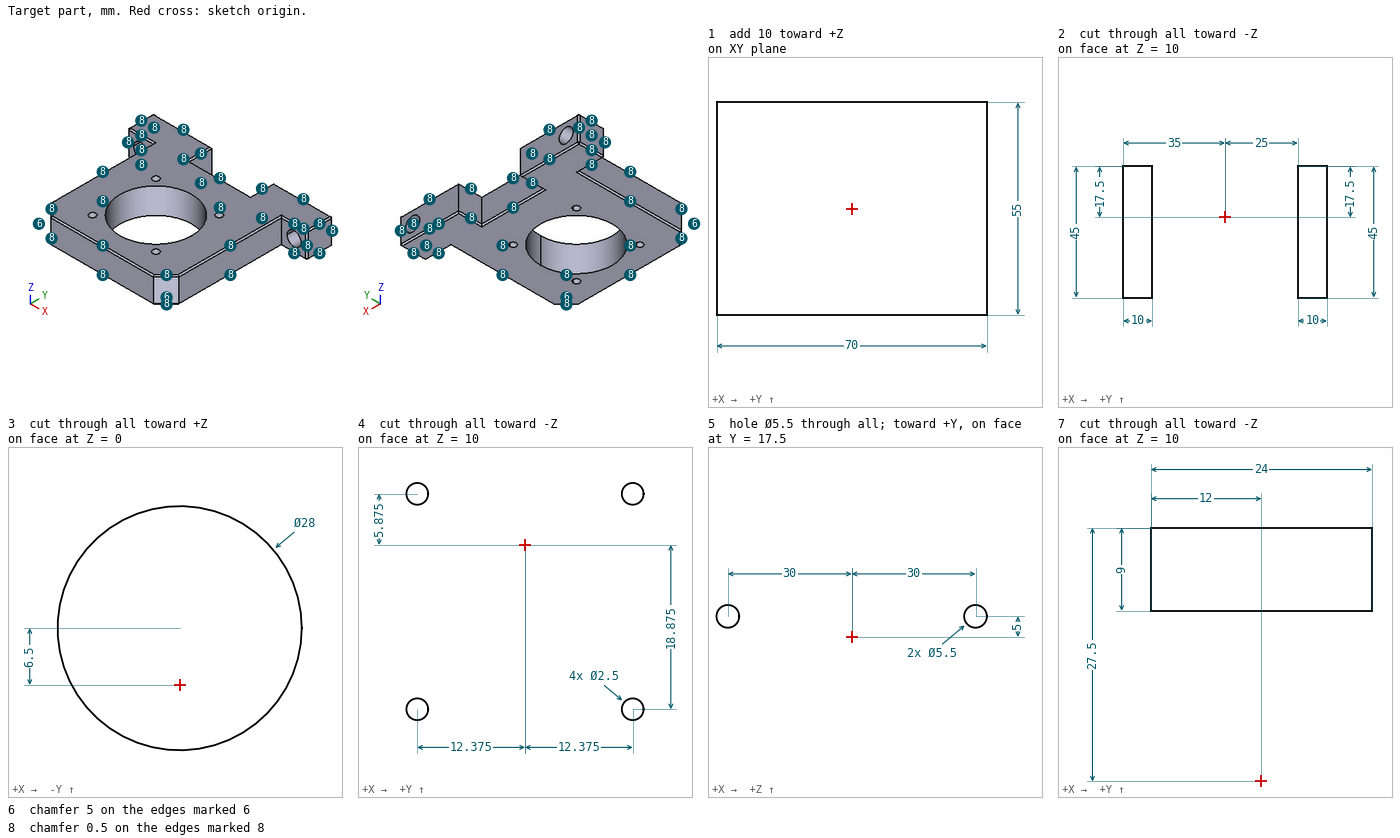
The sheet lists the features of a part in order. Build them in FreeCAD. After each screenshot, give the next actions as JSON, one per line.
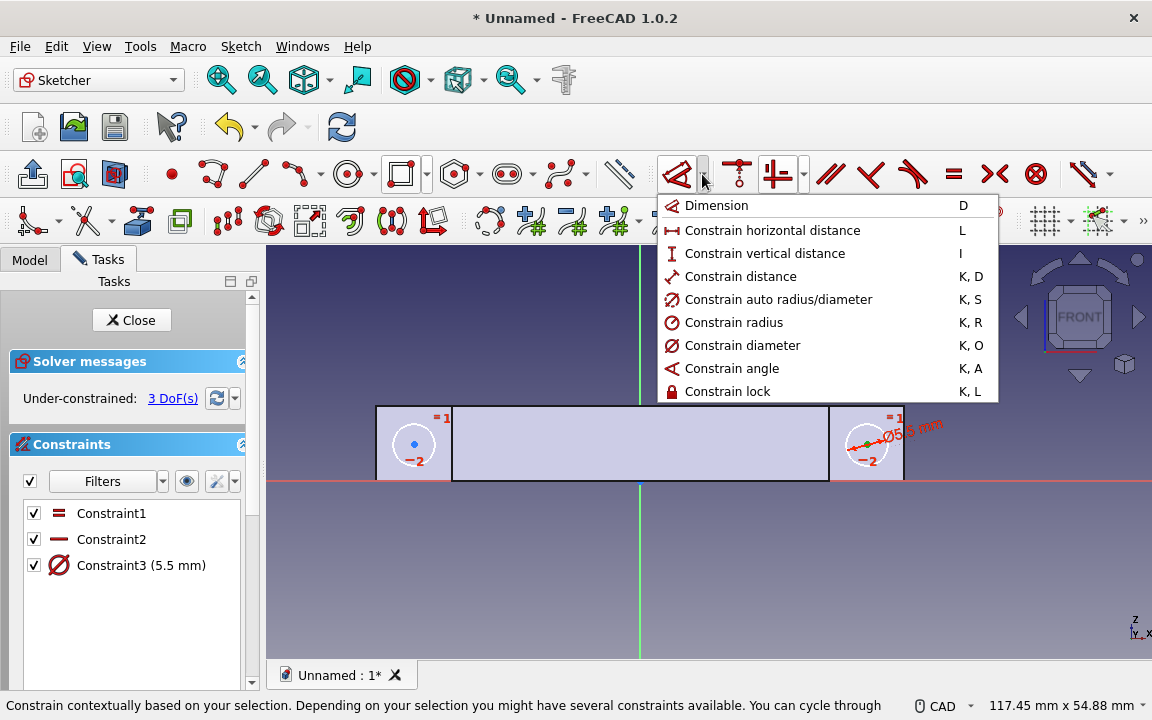
{"action": "left_click", "coordinate": [828, 254]}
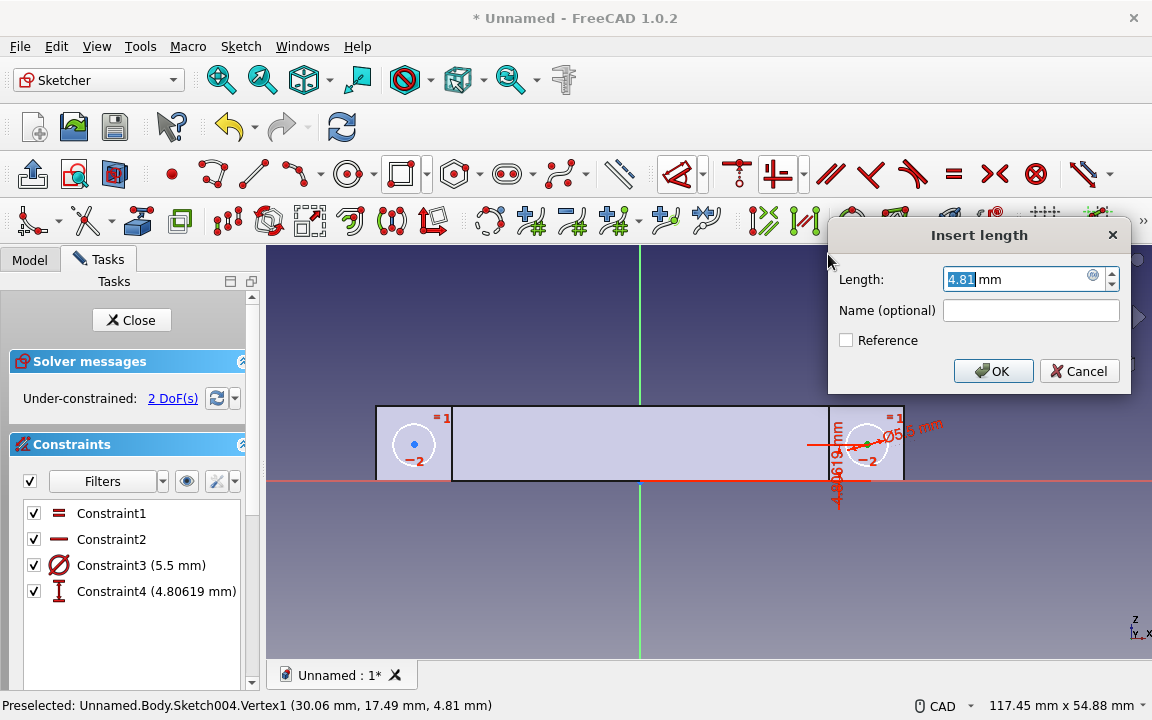
{"action": "type", "text": "5"}
{"action": "key", "text": "Return"}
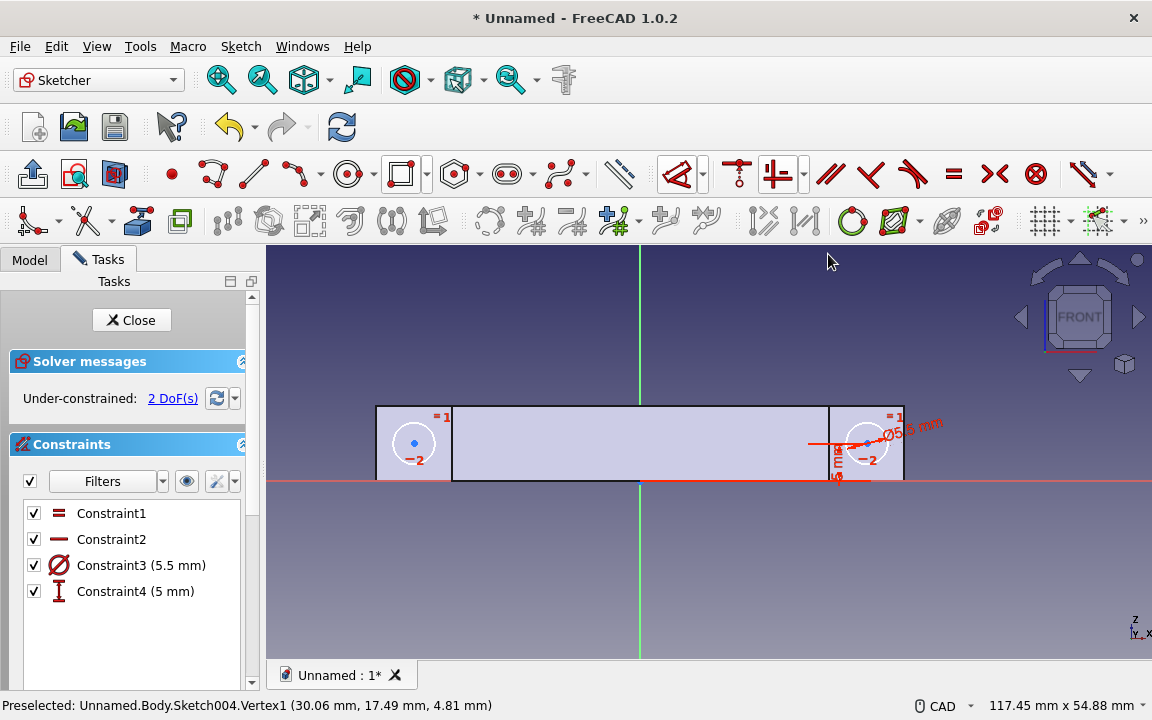
{"action": "left_click", "coordinate": [867, 444]}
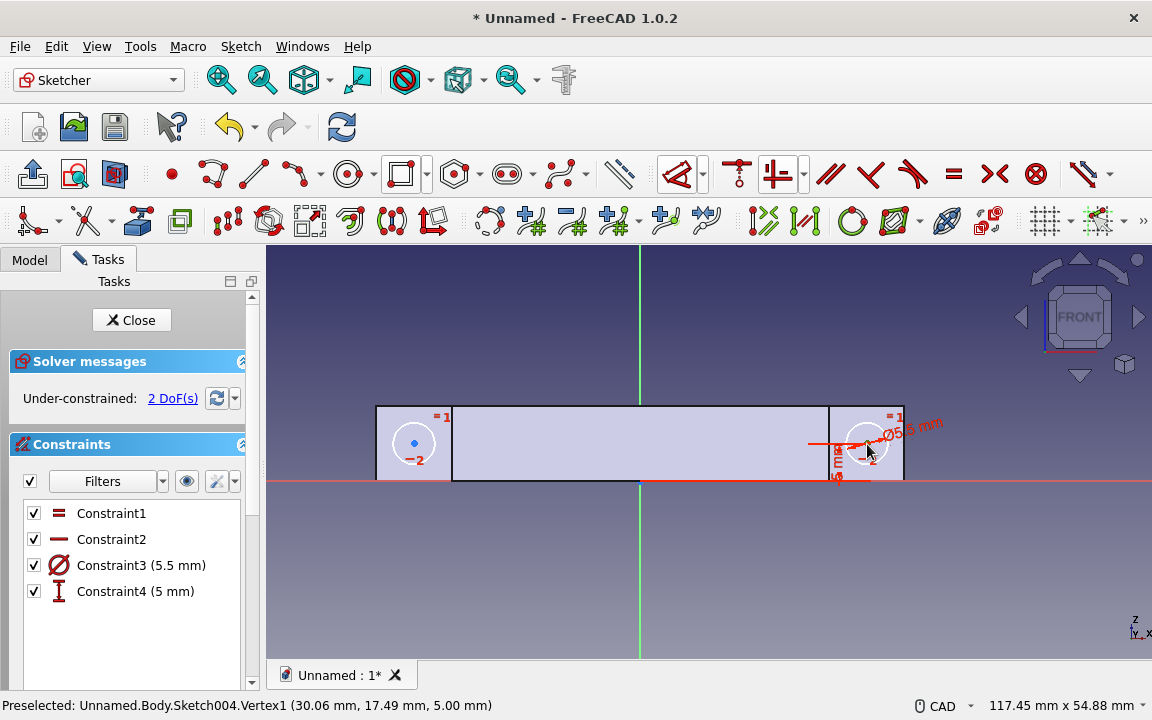
{"action": "key", "text": "l"}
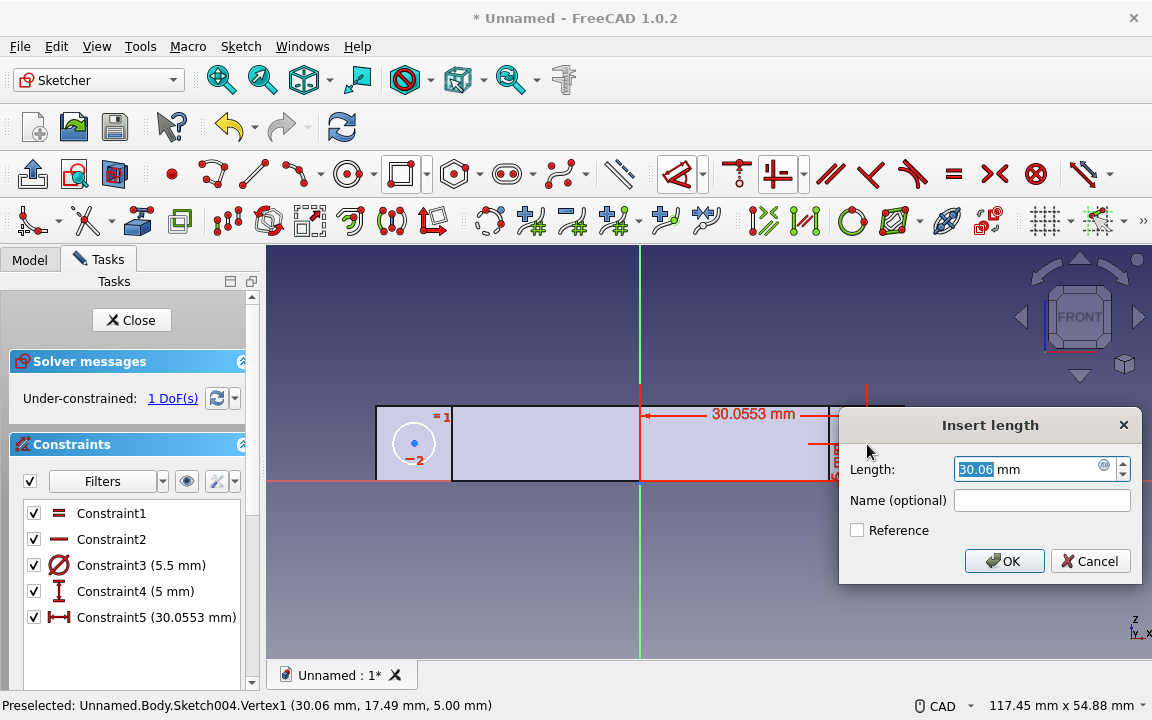
{"action": "type", "text": "30"}
{"action": "key", "text": "Return"}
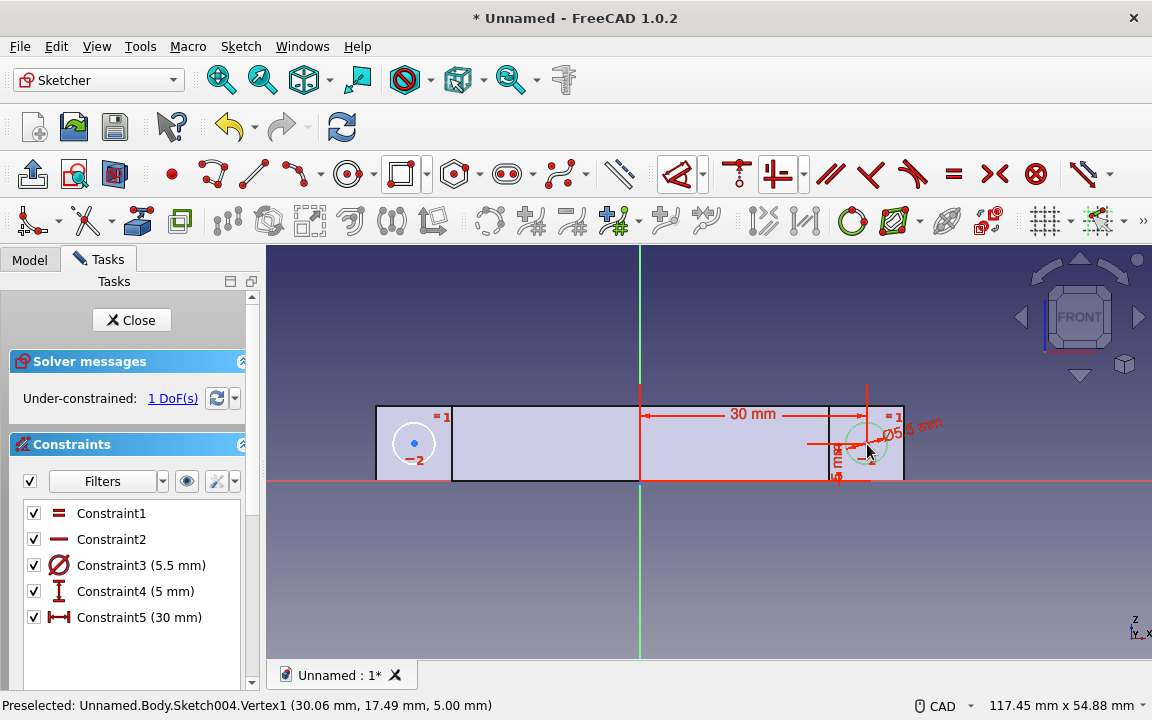
{"action": "left_click", "coordinate": [414, 444]}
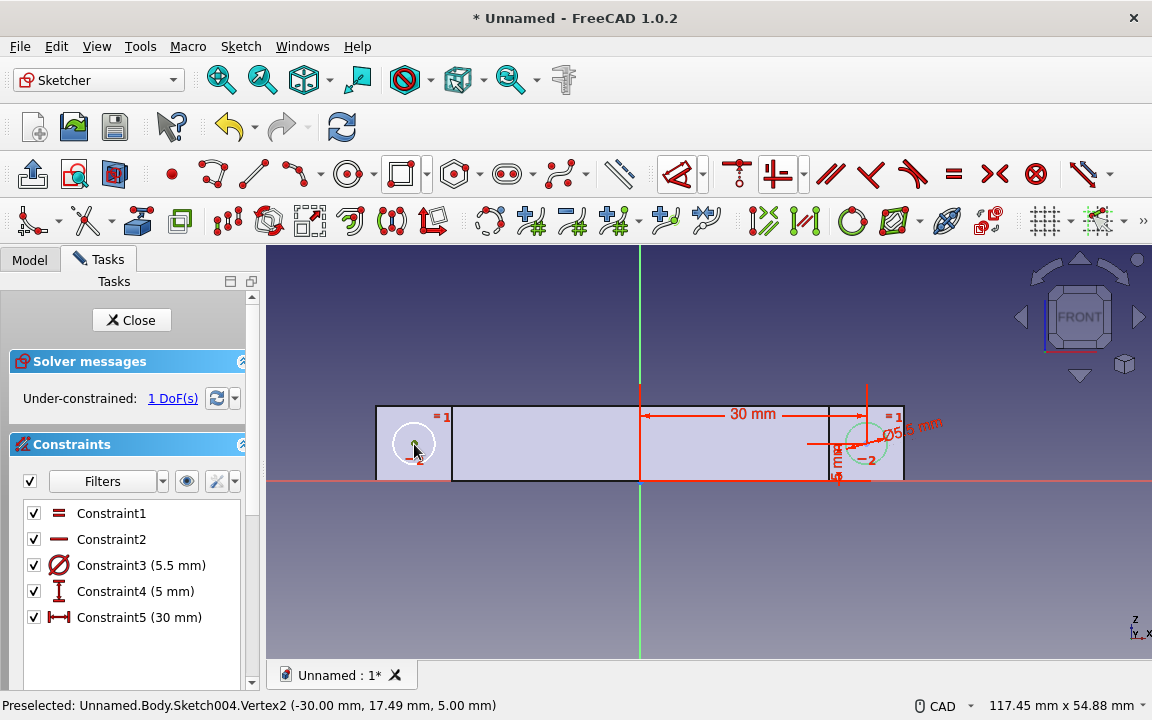
{"action": "left_click", "coordinate": [702, 174]}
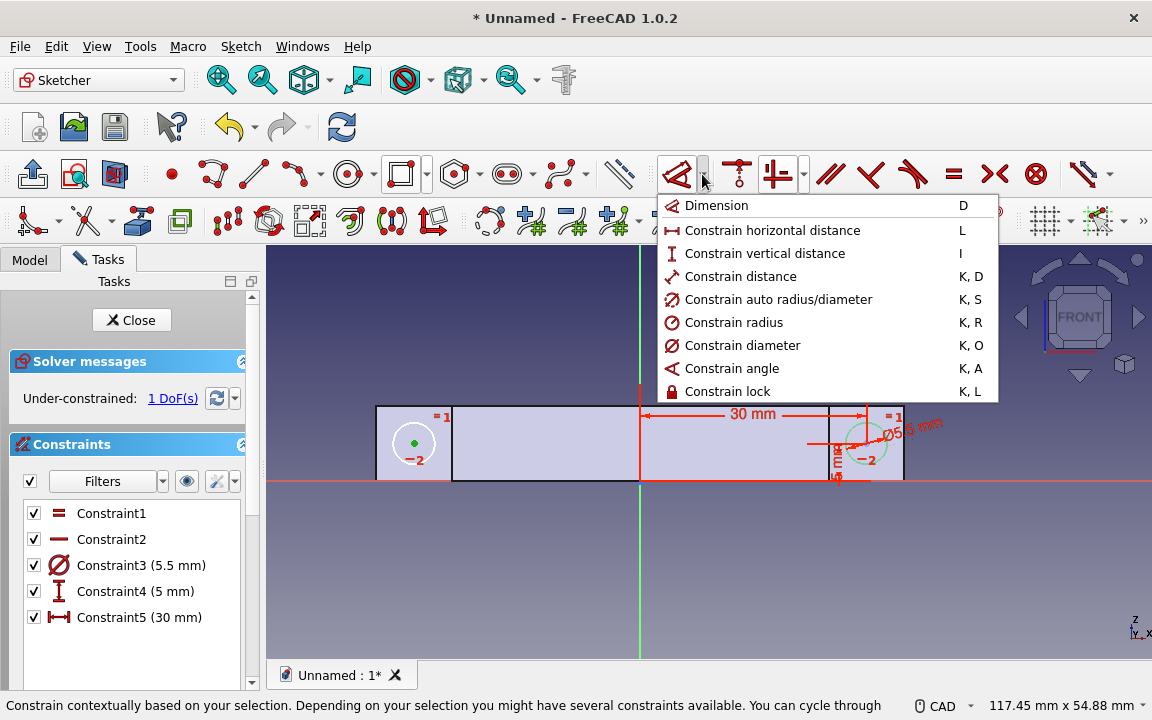
{"action": "left_click", "coordinate": [828, 230]}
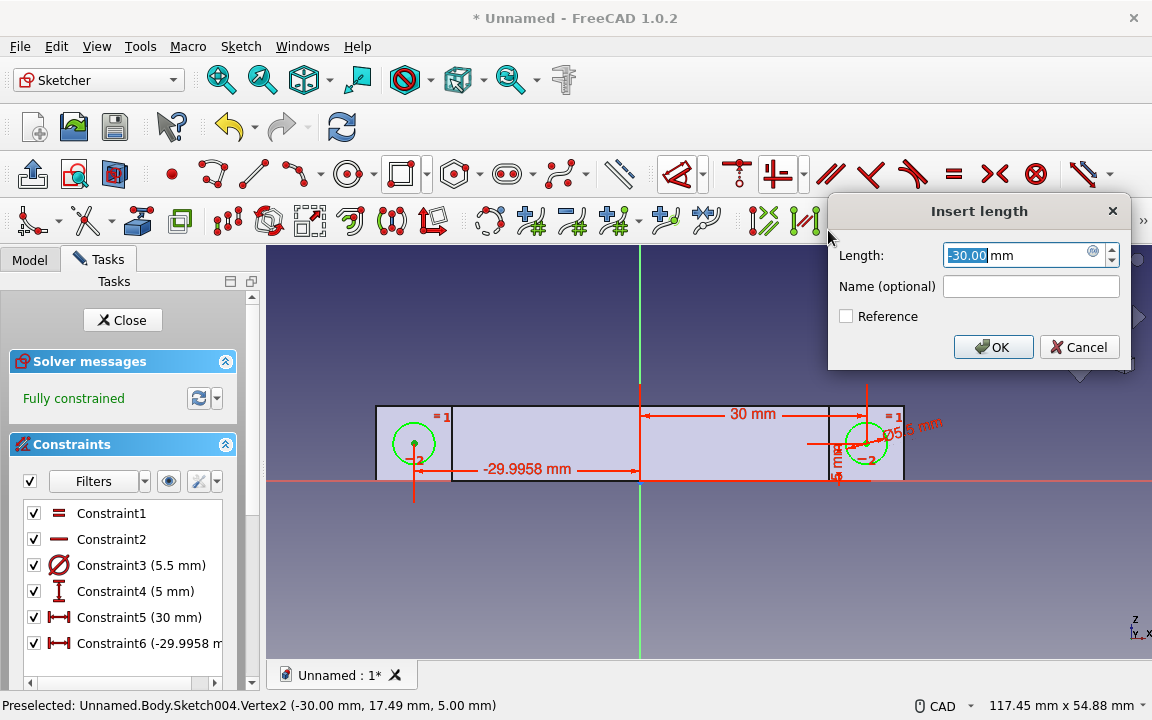
{"action": "type", "text": "-30"}
{"action": "key", "text": "Return"}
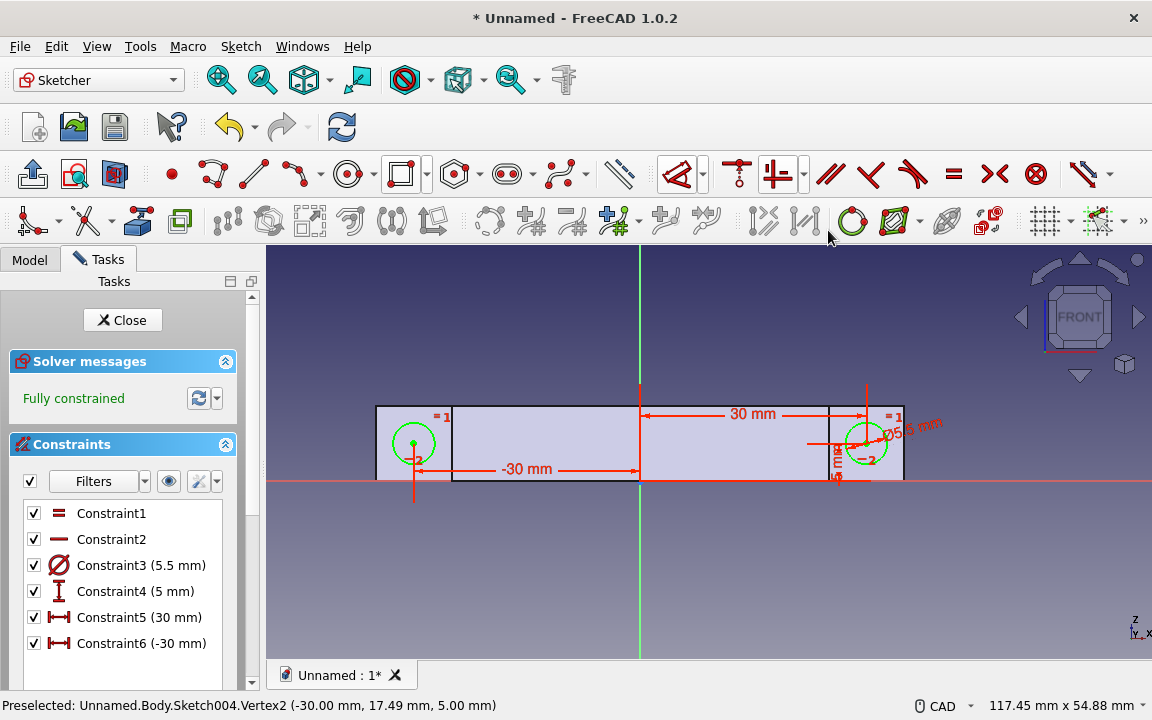
{"action": "left_click", "coordinate": [123, 320]}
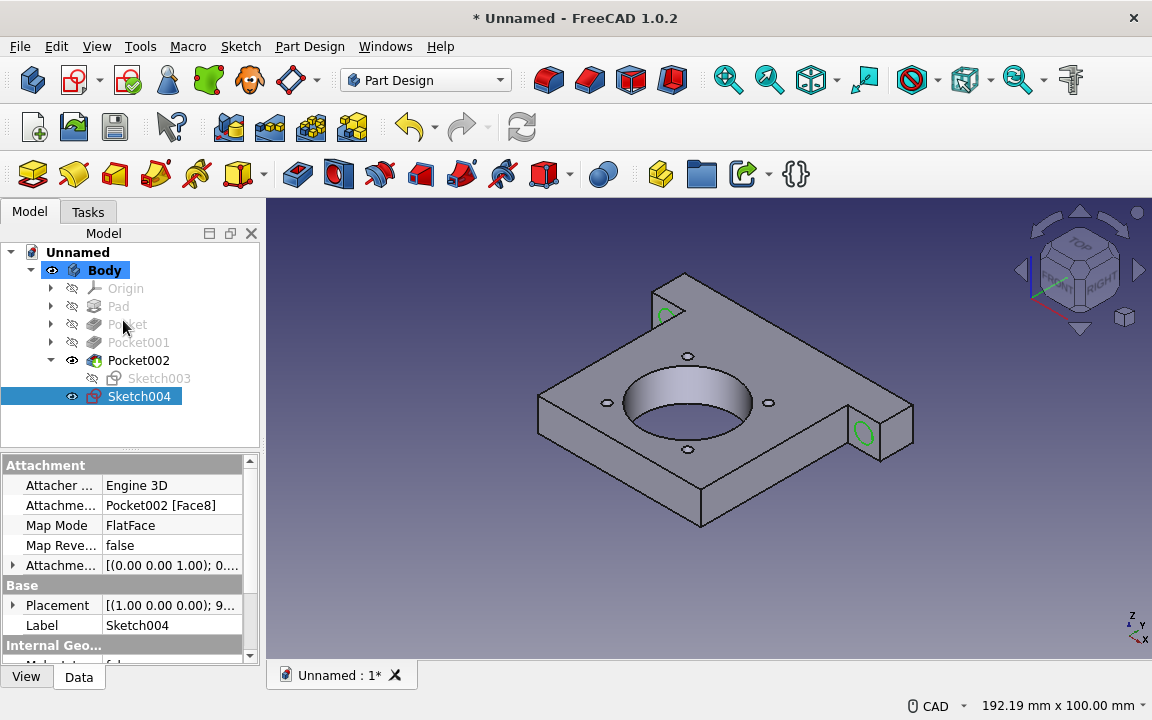
{"action": "left_click", "coordinate": [339, 174]}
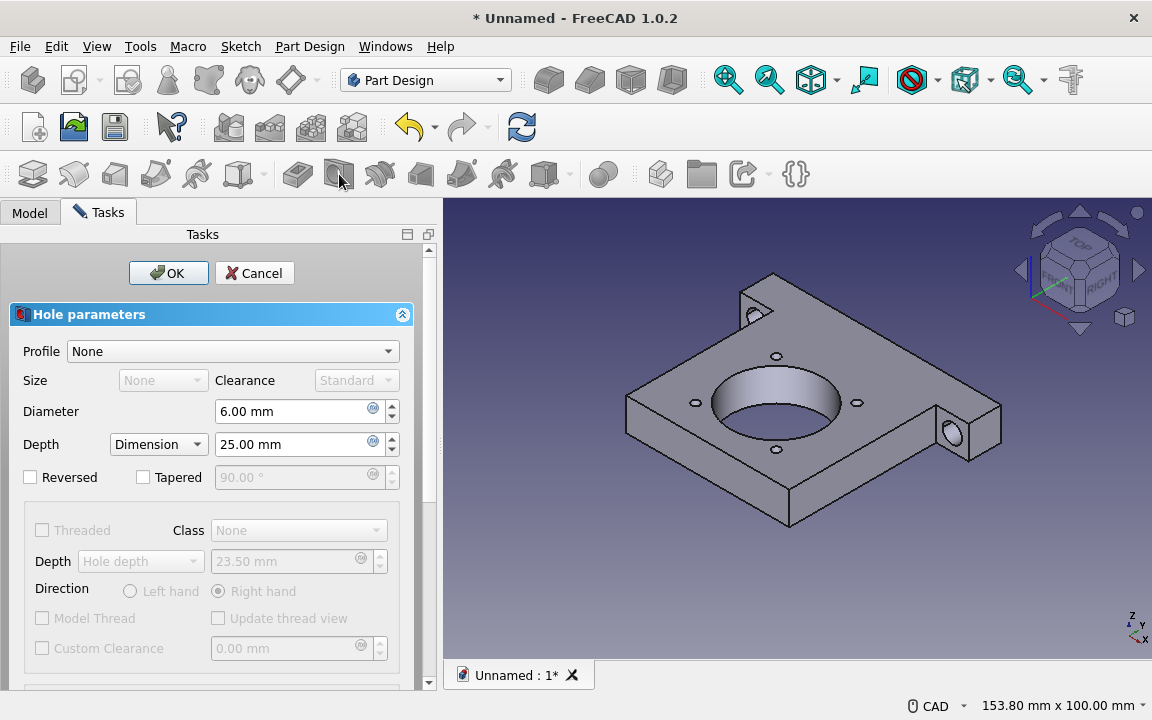
{"action": "triple_click", "coordinate": [300, 412]}